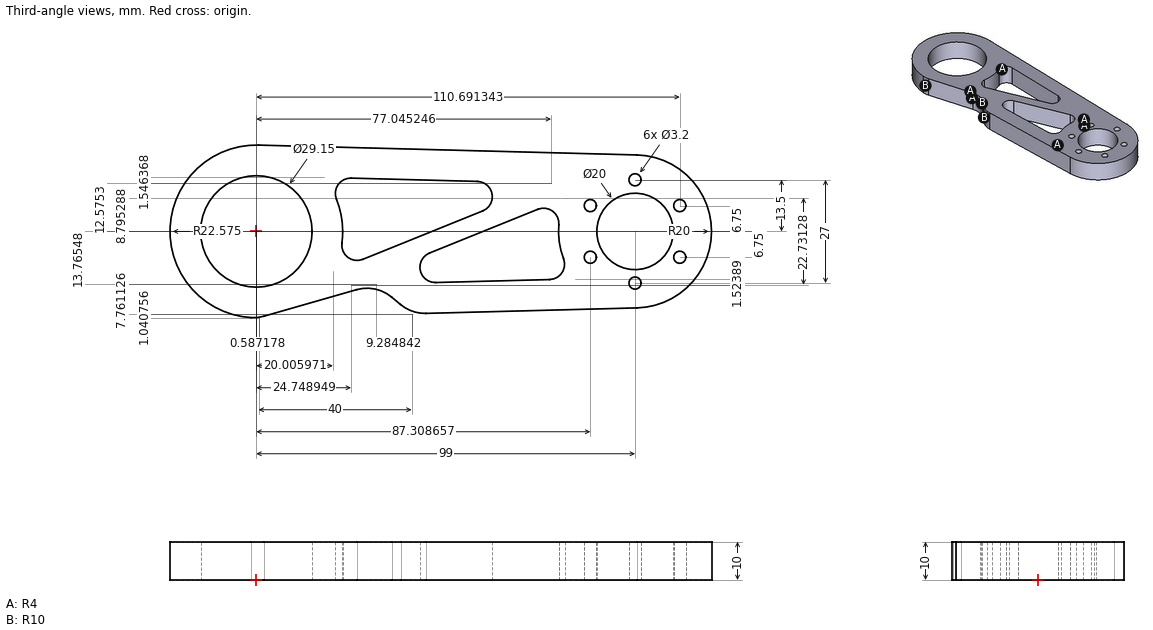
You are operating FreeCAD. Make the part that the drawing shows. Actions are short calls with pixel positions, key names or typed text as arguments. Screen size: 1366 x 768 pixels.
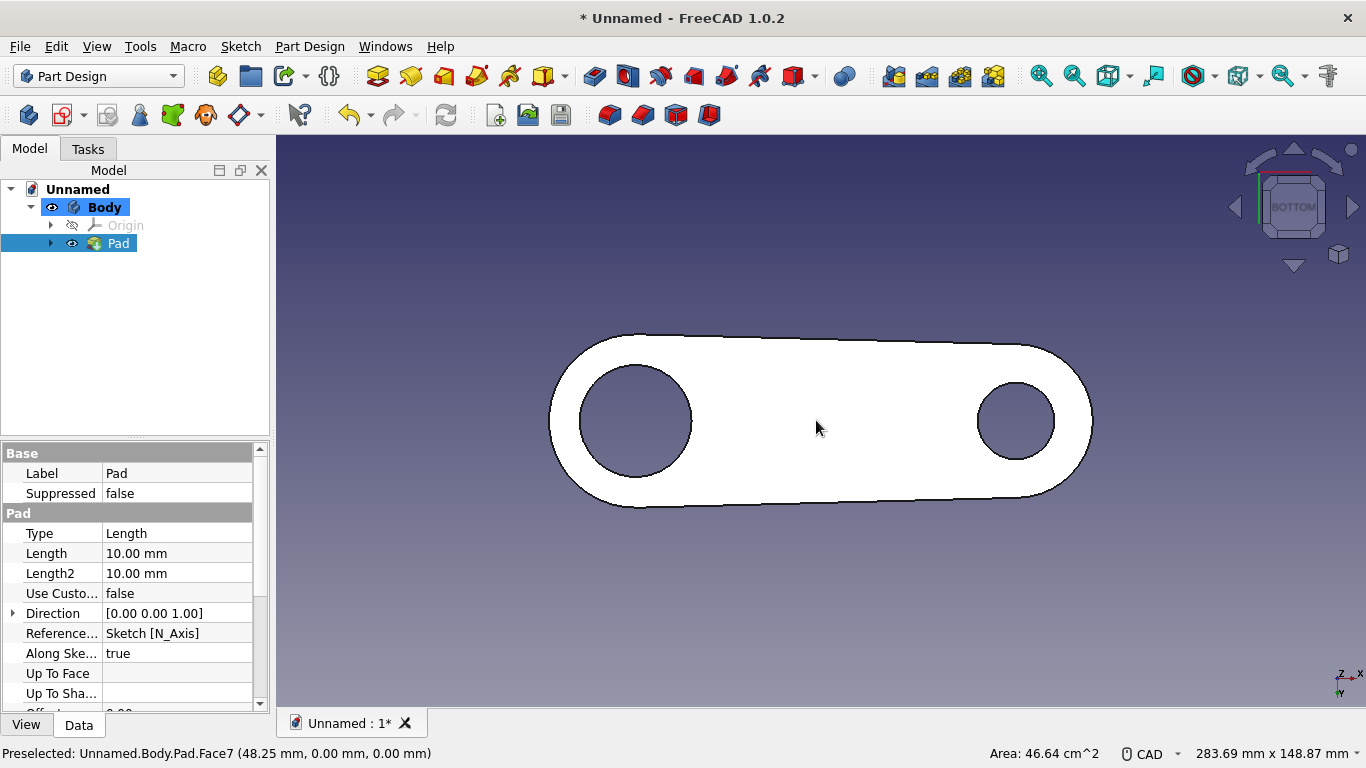
click(62, 116)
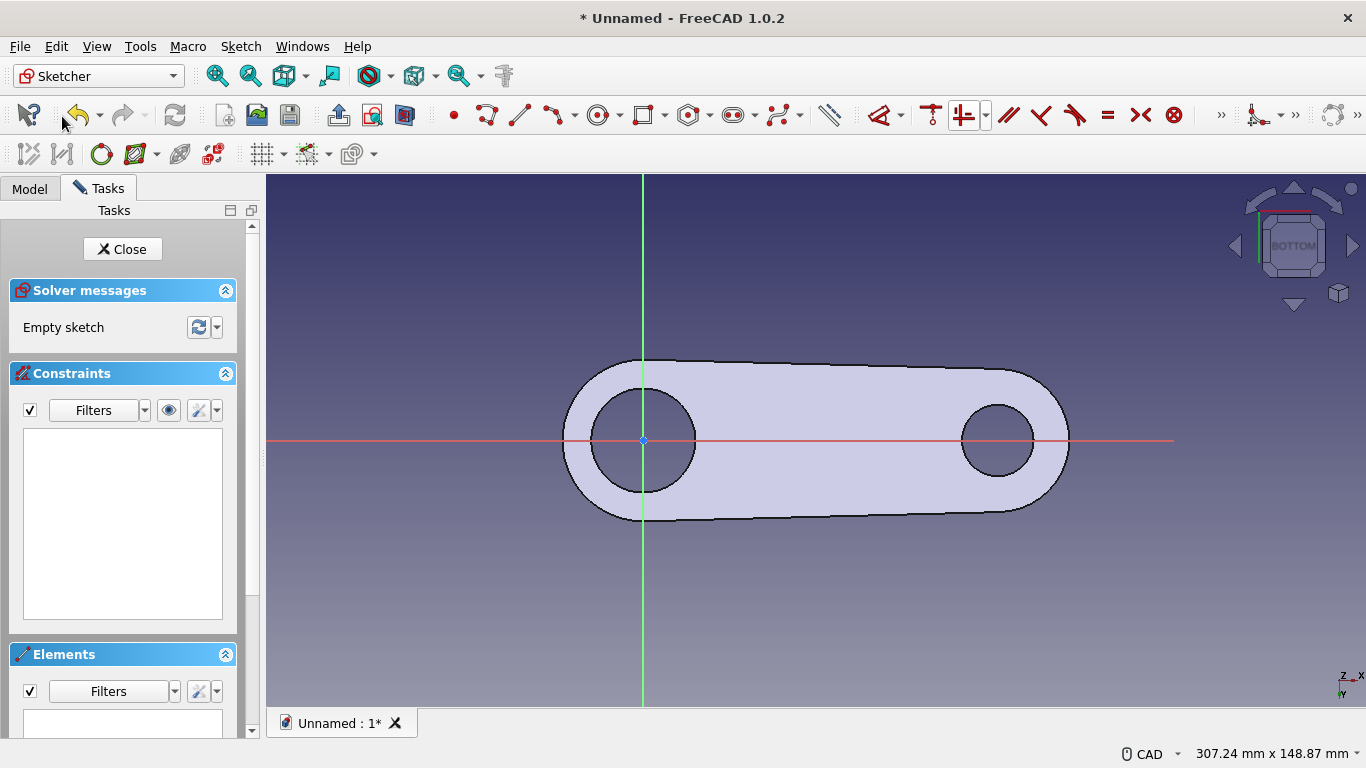
scroll(829, 441, up, 4)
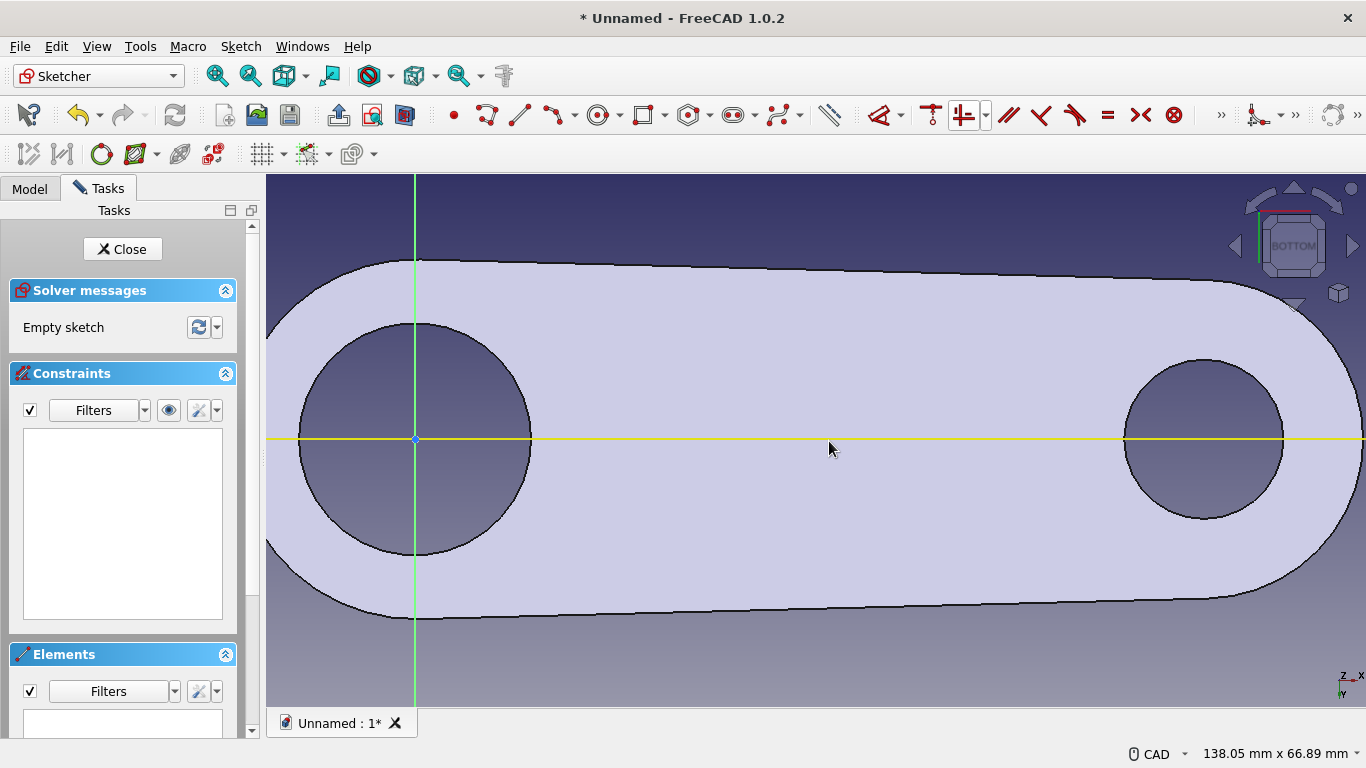
key(g)
key(m)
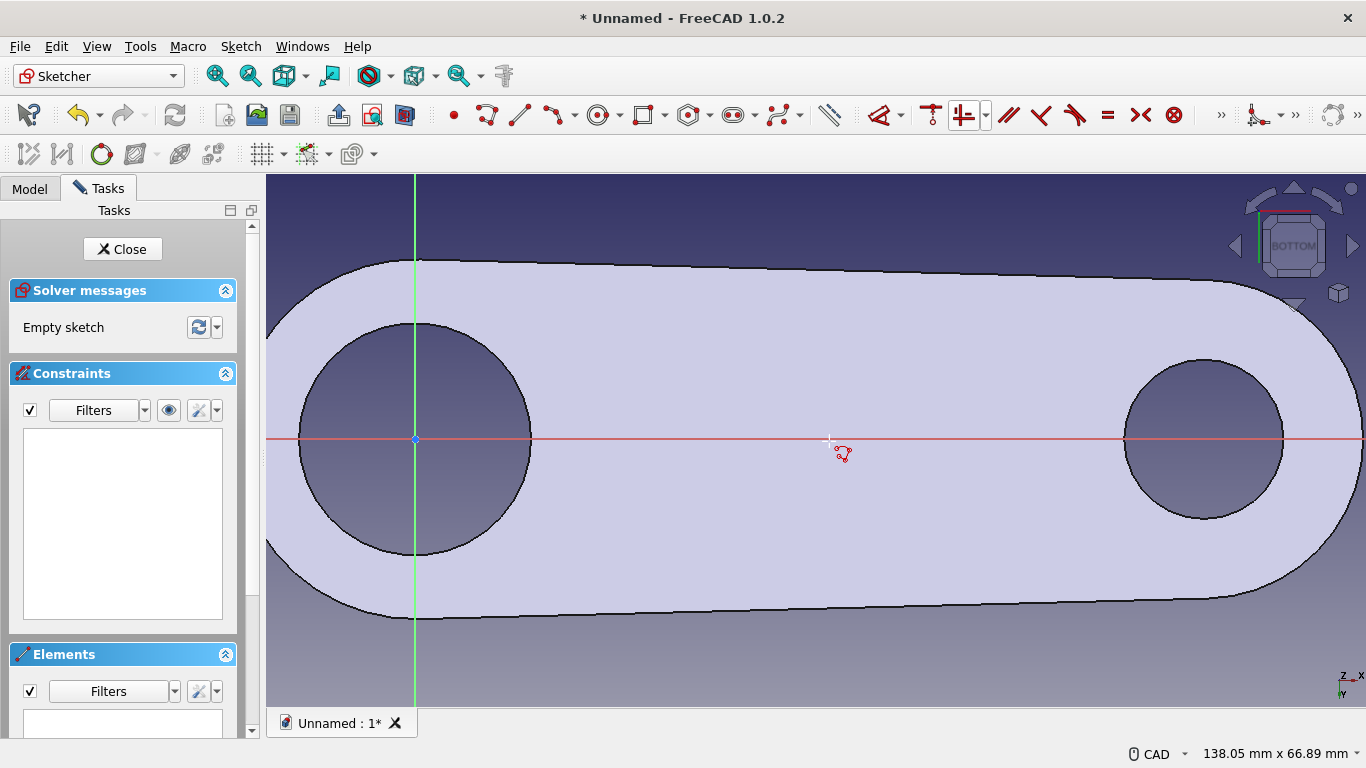
click(574, 356)
click(1029, 539)
click(555, 562)
right_click(555, 562)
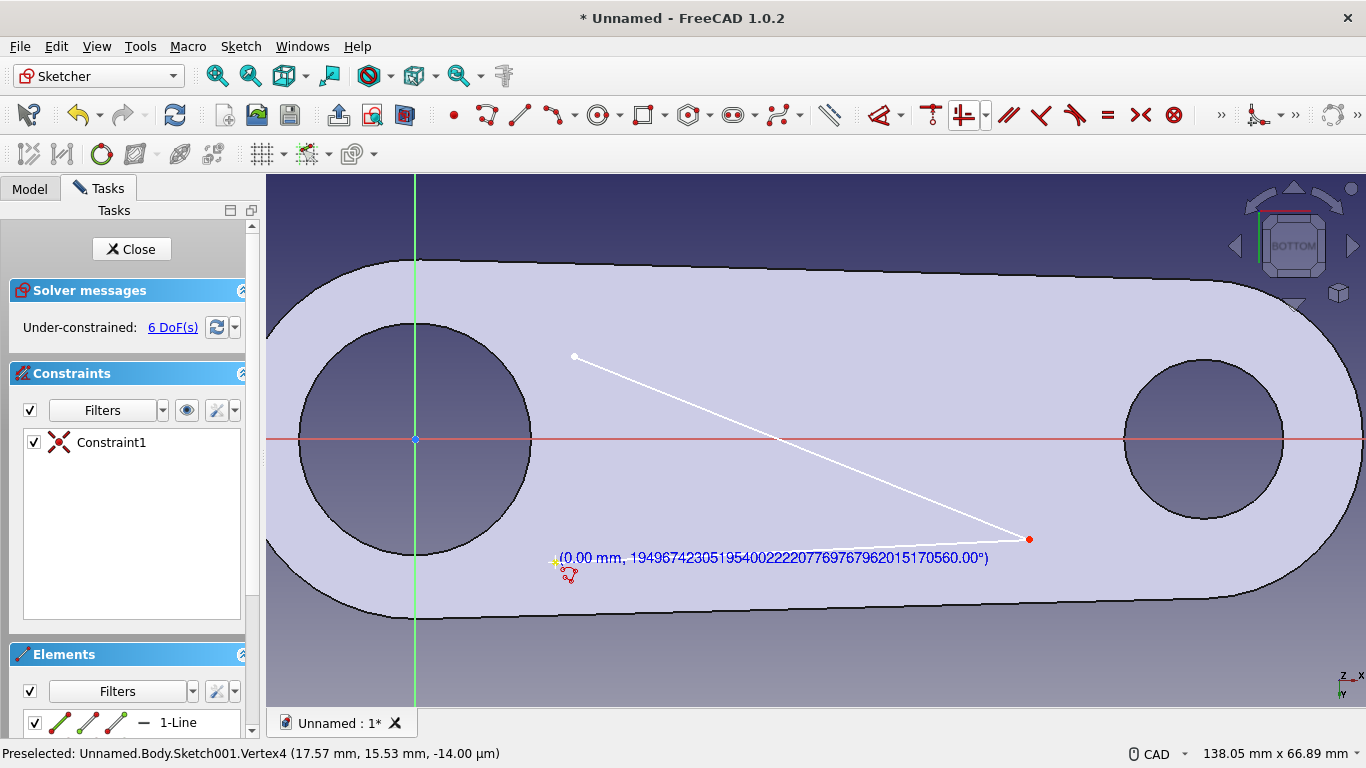
key(g)
key(3)
key(a)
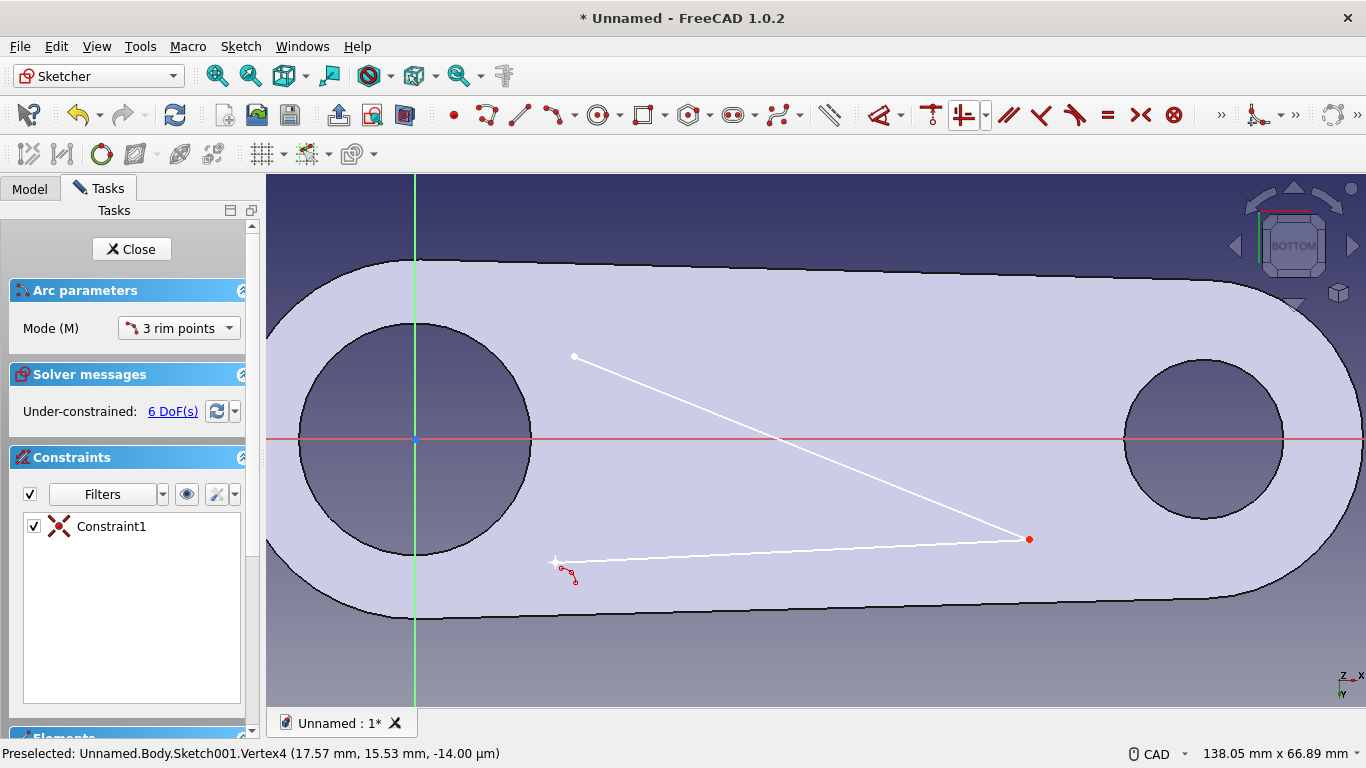
click(555, 563)
click(574, 357)
click(594, 457)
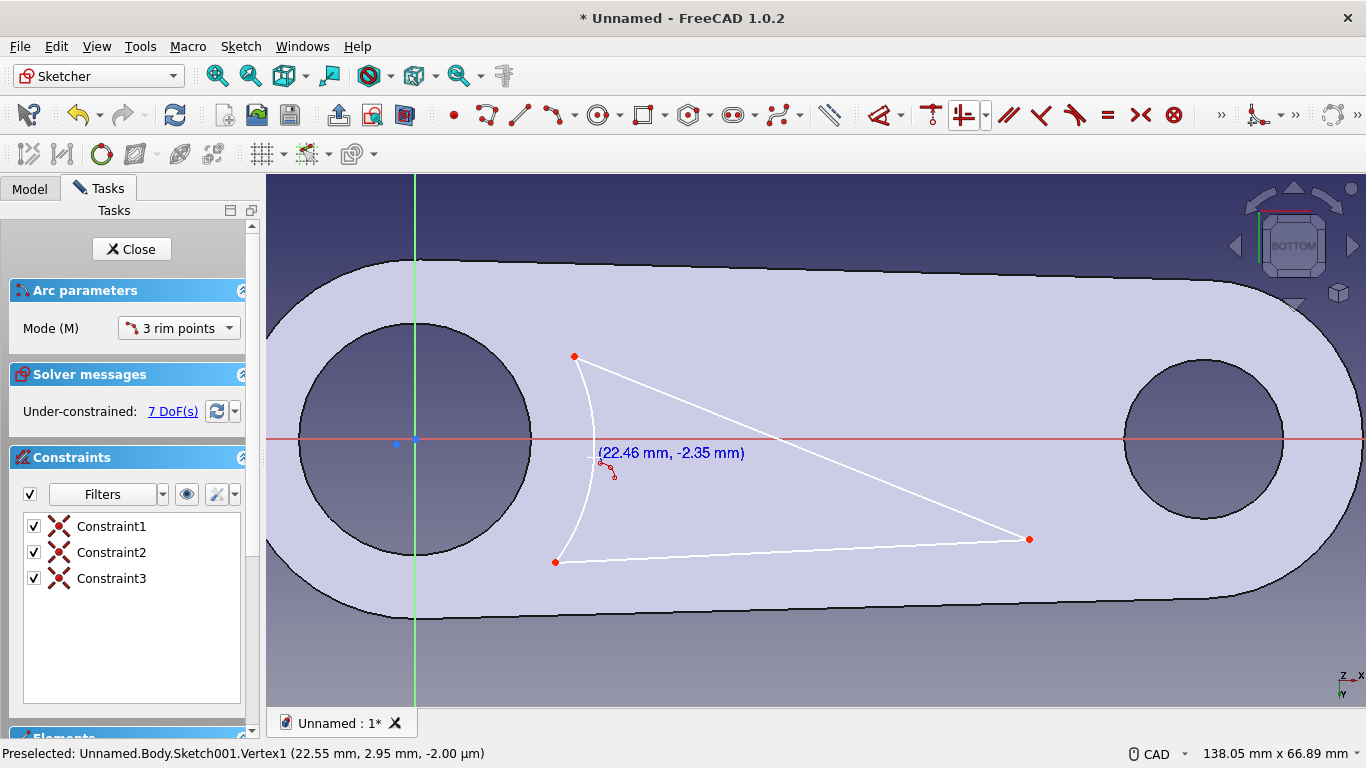
click(487, 116)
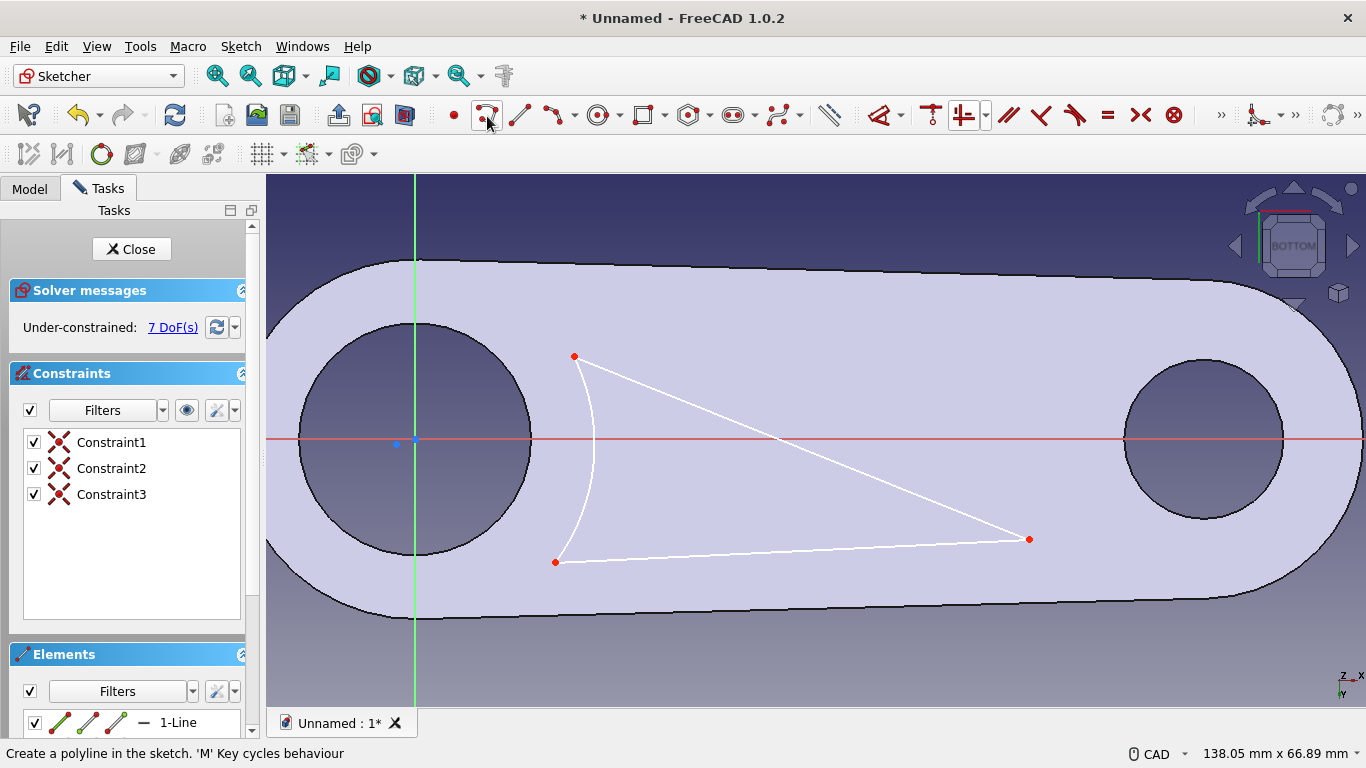
click(1061, 509)
click(612, 328)
click(1079, 351)
right_click(1079, 351)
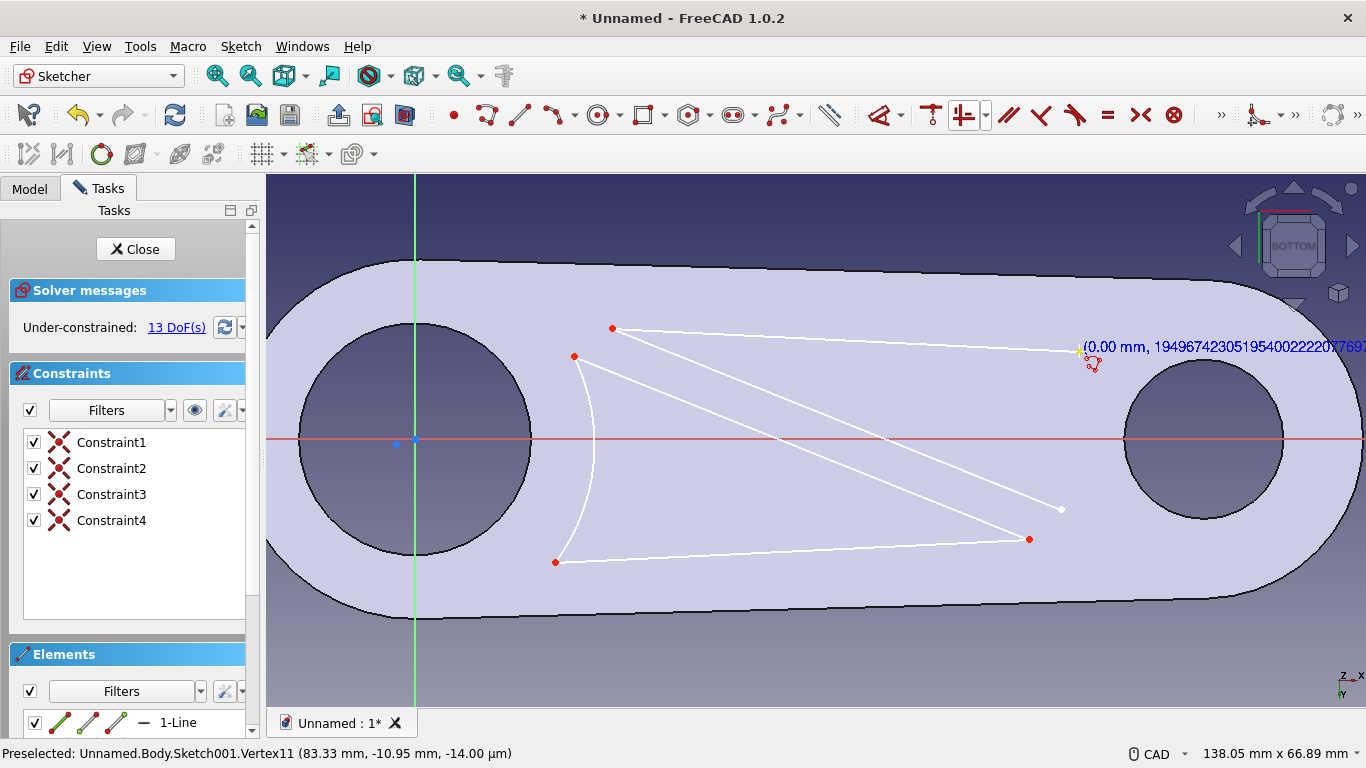
click(552, 116)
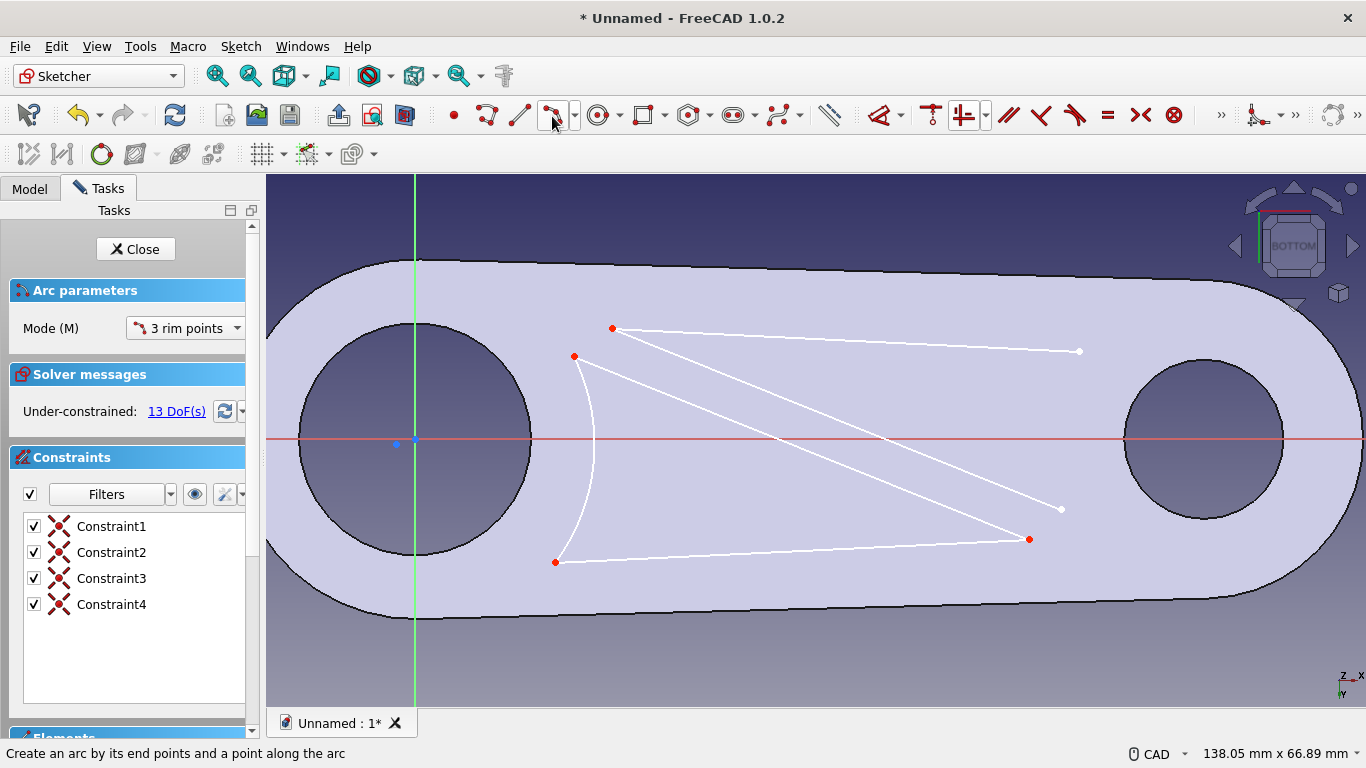
click(1079, 352)
click(1061, 510)
click(1045, 422)
key(Escape)